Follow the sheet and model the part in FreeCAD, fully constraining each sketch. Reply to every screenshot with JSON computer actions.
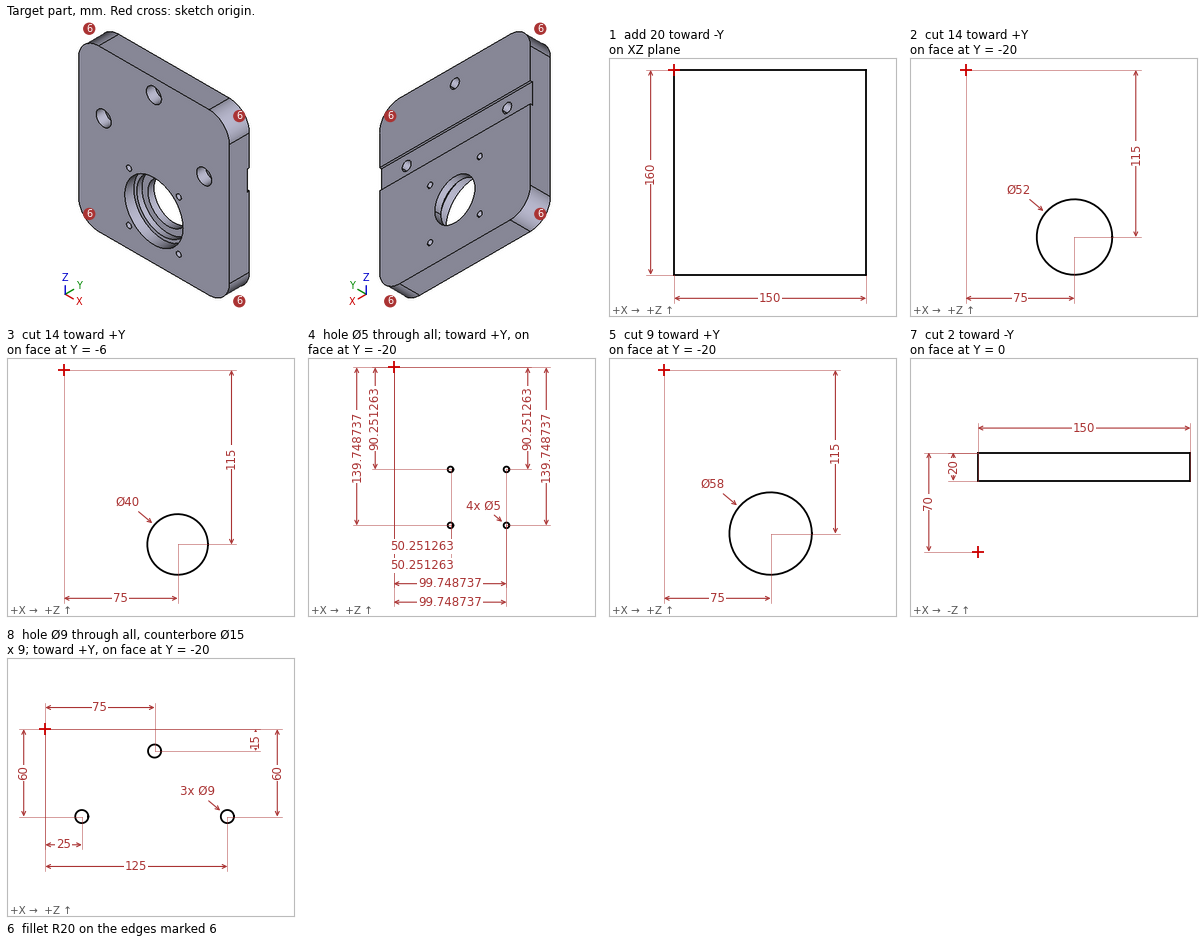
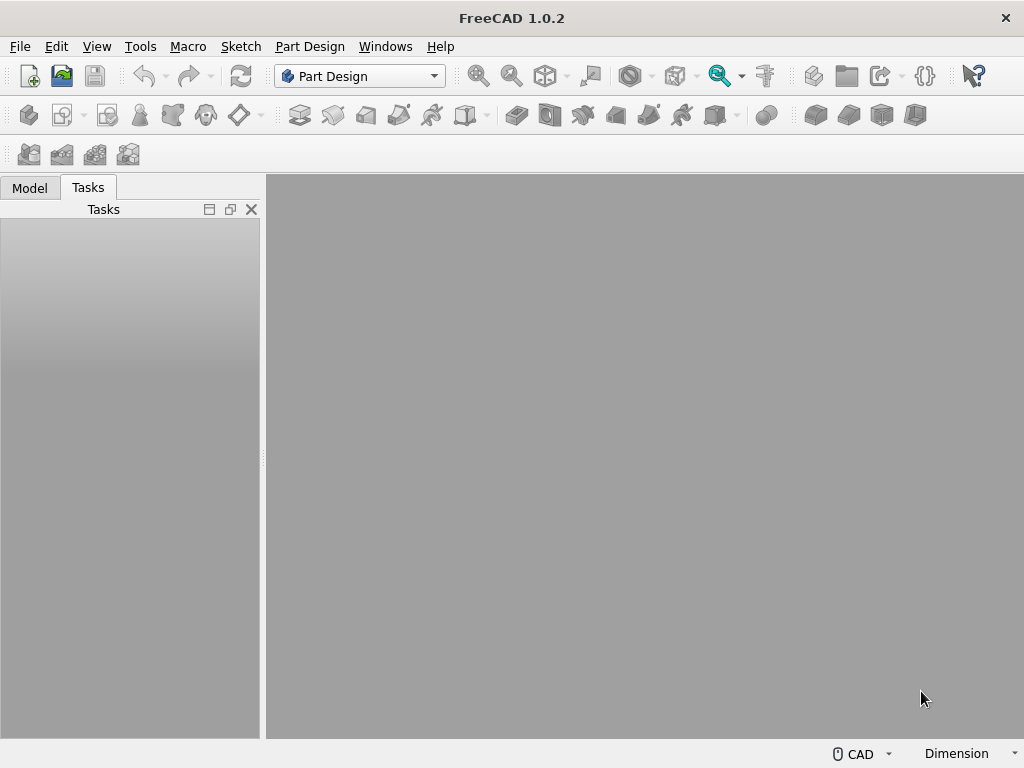
{"action": "left_click", "coordinate": [29, 76]}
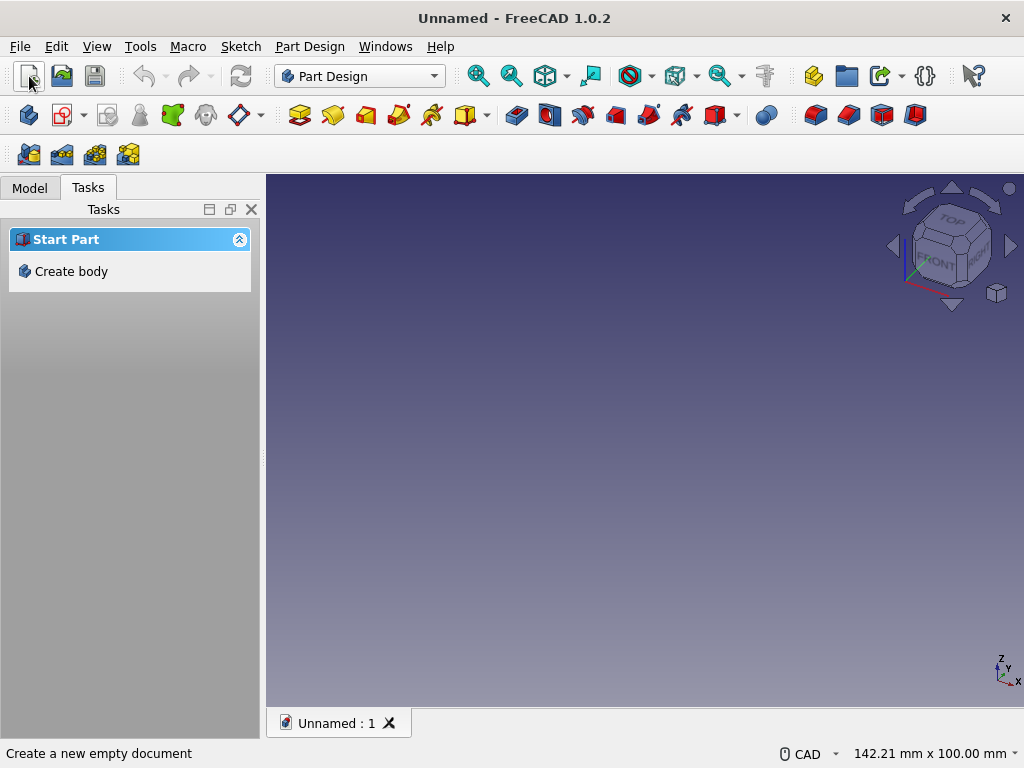
{"action": "left_click", "coordinate": [62, 116]}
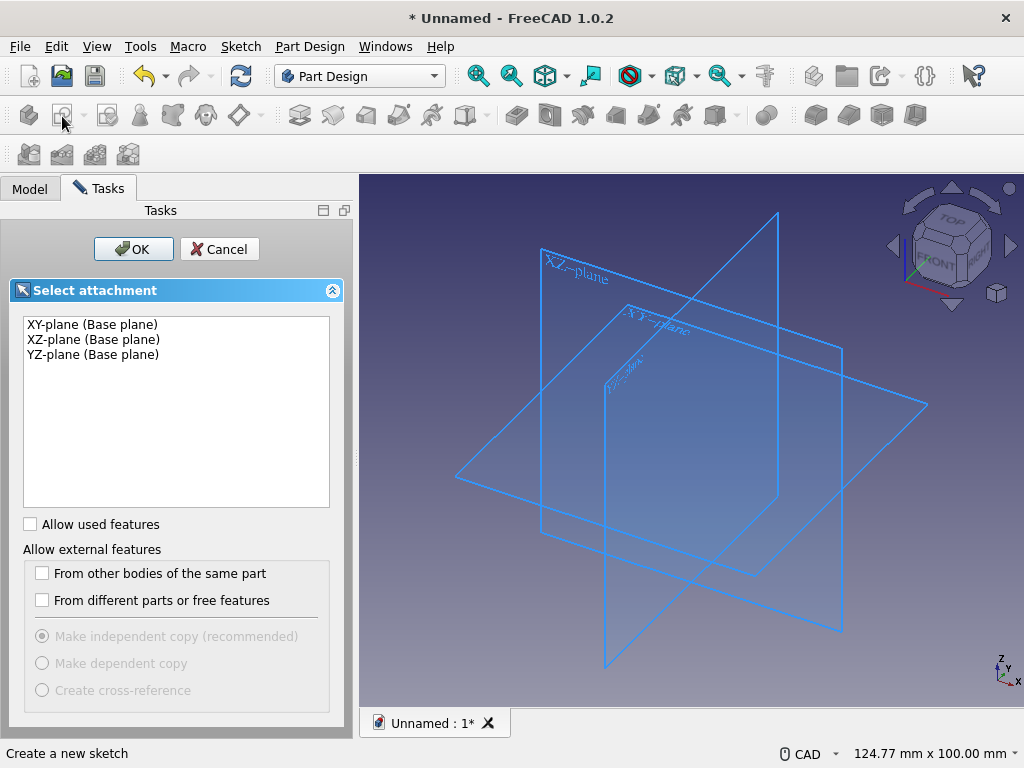
{"action": "left_click", "coordinate": [84, 340]}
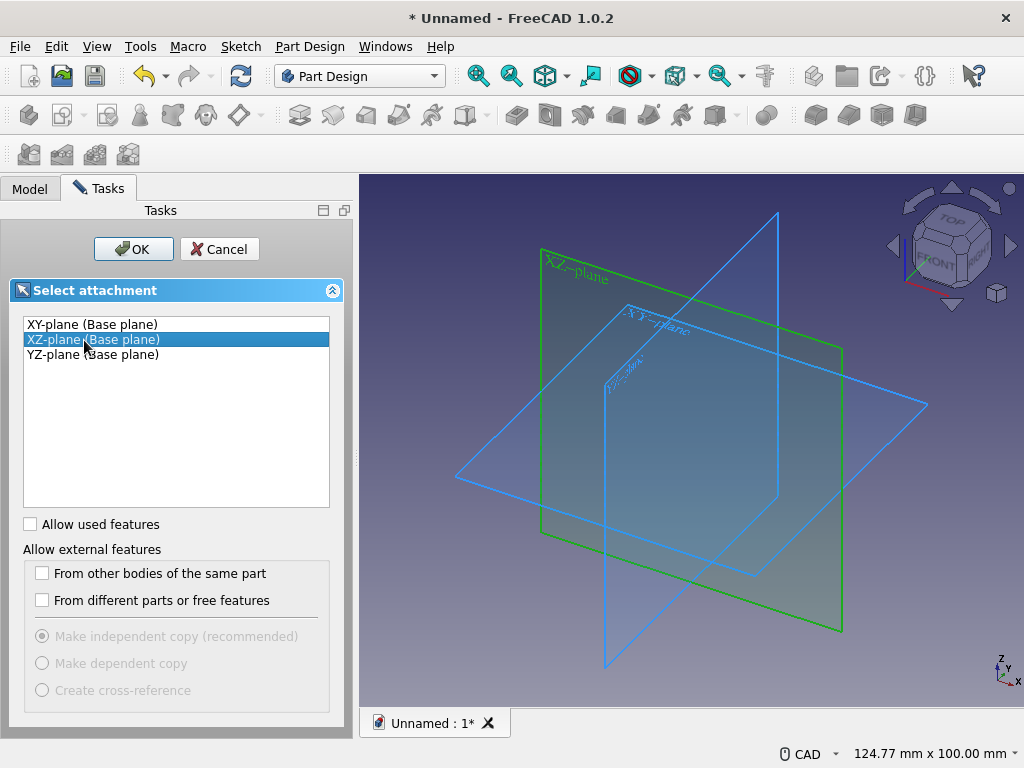
{"action": "left_click", "coordinate": [134, 249]}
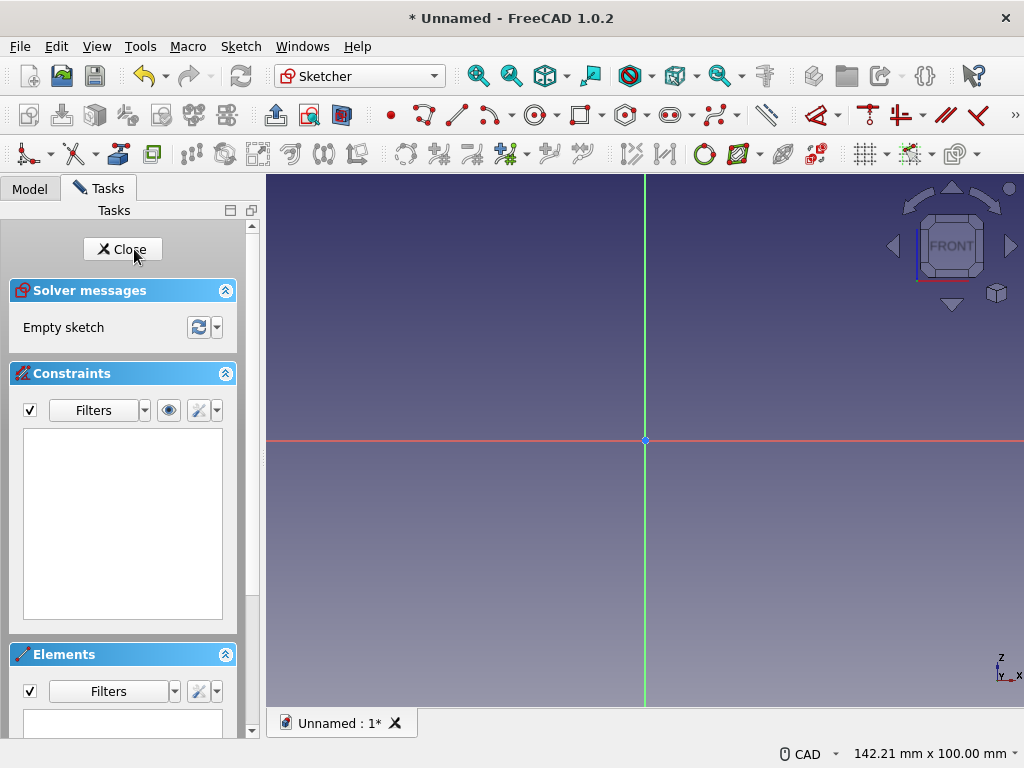
{"action": "scroll", "coordinate": [304, 202], "scroll_direction": "down", "scroll_amount": 5}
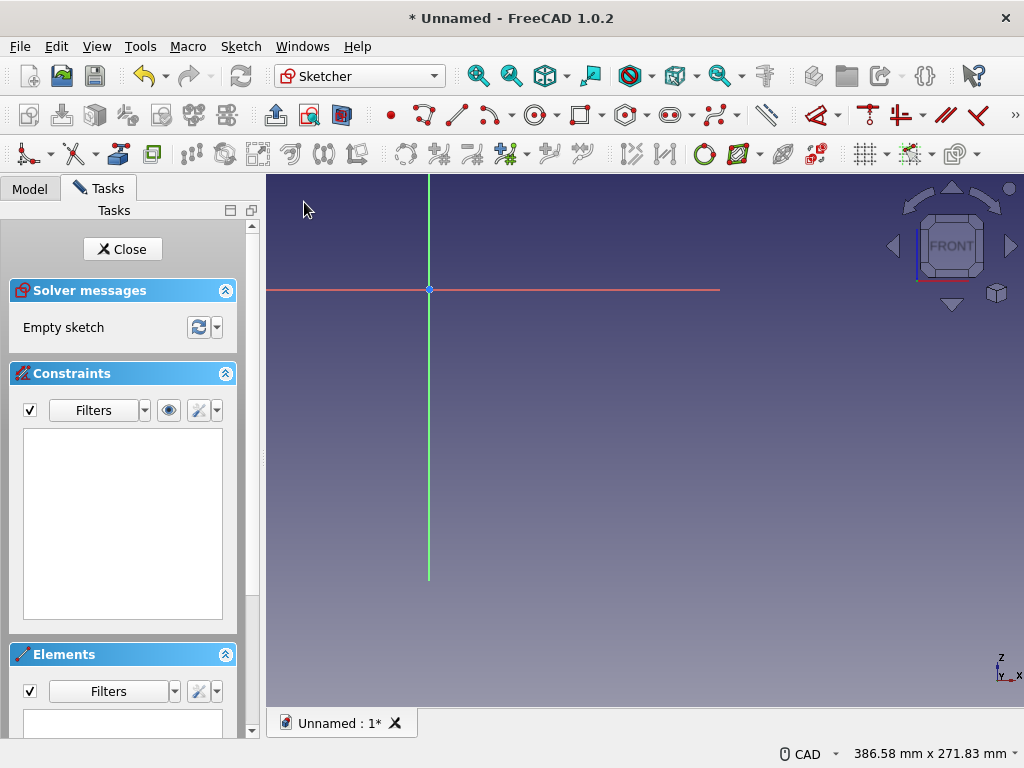
{"action": "left_click", "coordinate": [580, 116]}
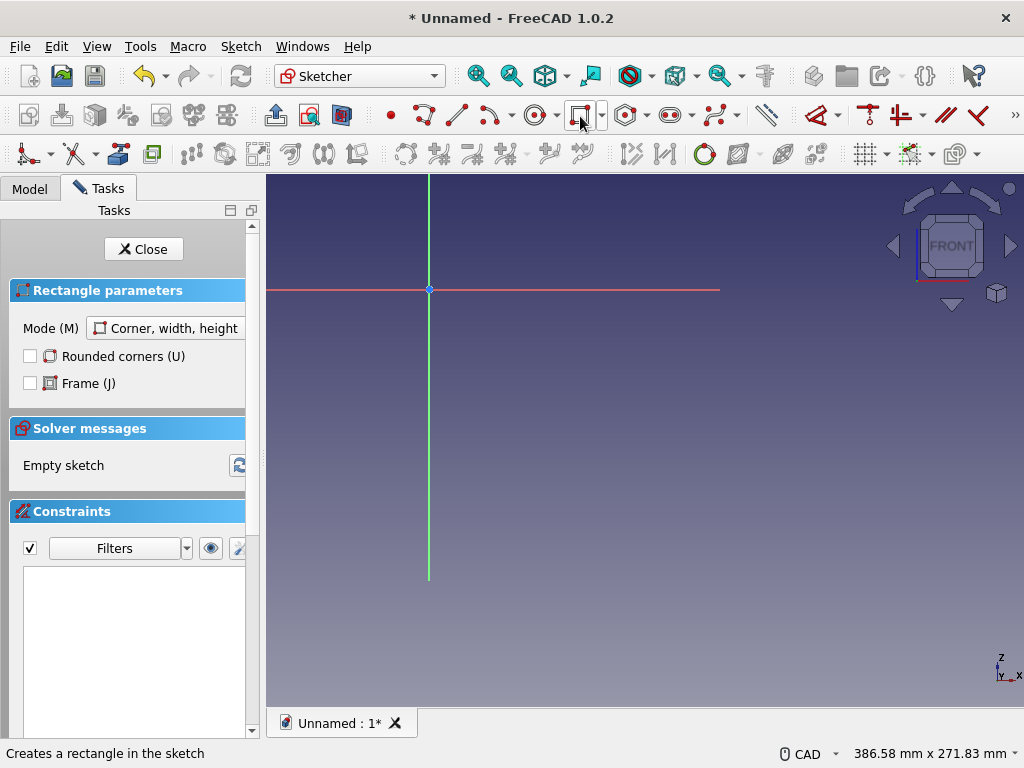
{"action": "left_click", "coordinate": [429, 290]}
{"action": "left_click", "coordinate": [724, 604]}
{"action": "key", "text": "Escape"}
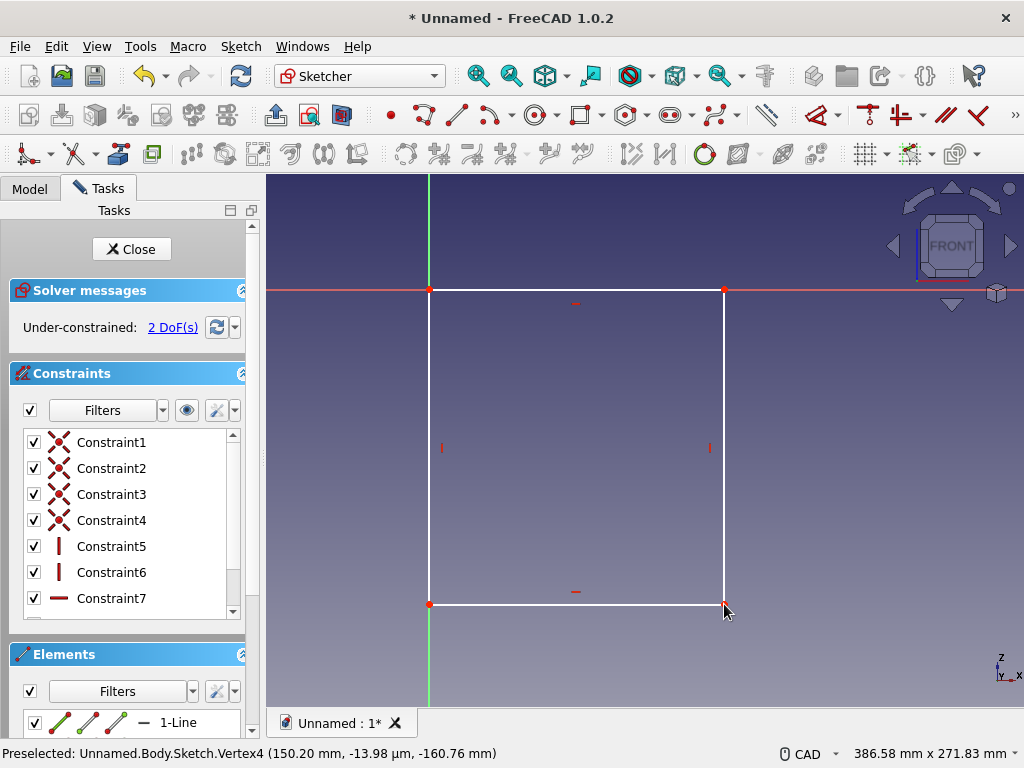
{"action": "left_click", "coordinate": [429, 384]}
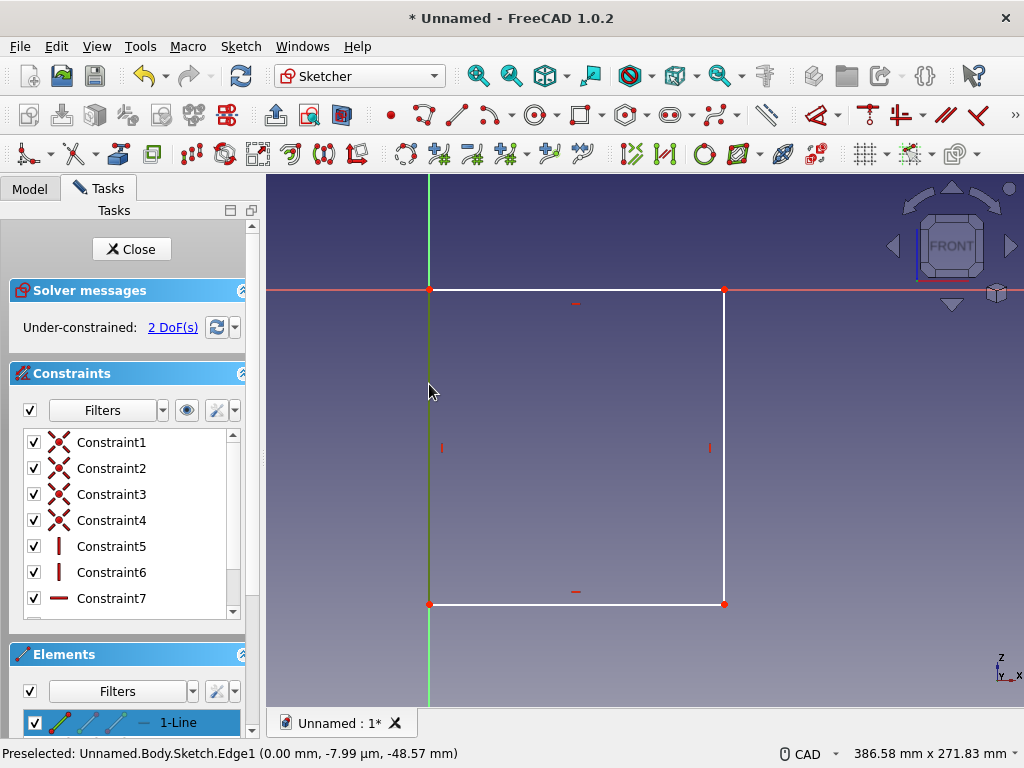
{"action": "key", "text": "i"}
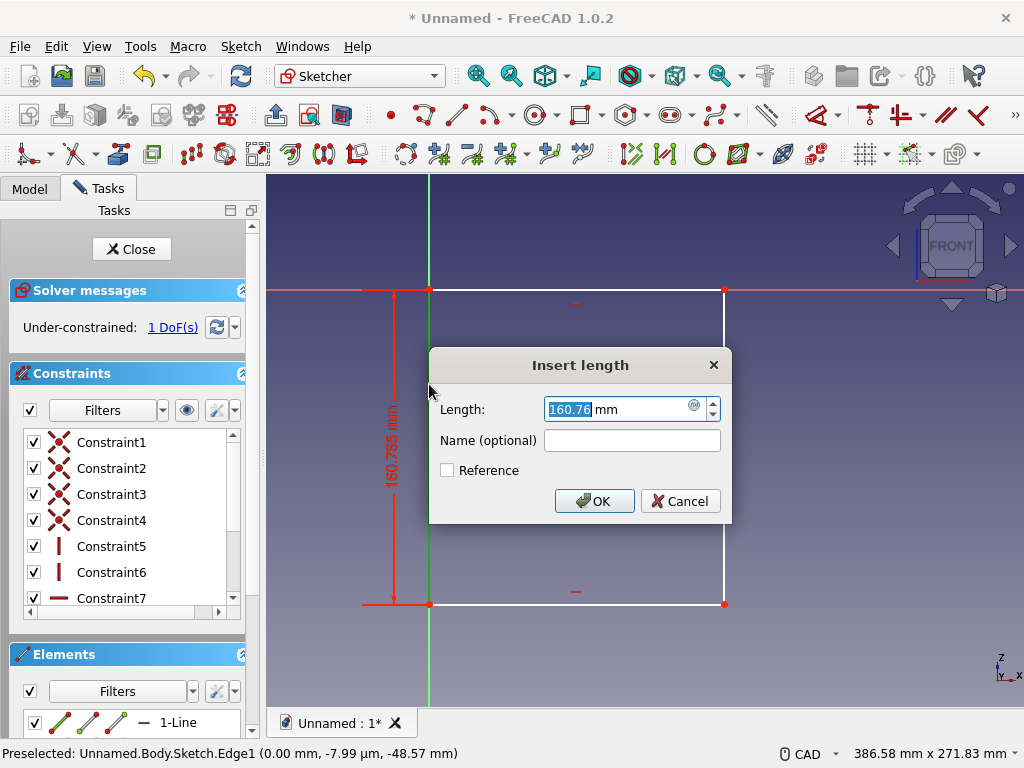
{"action": "type", "text": "160"}
{"action": "key", "text": "Return"}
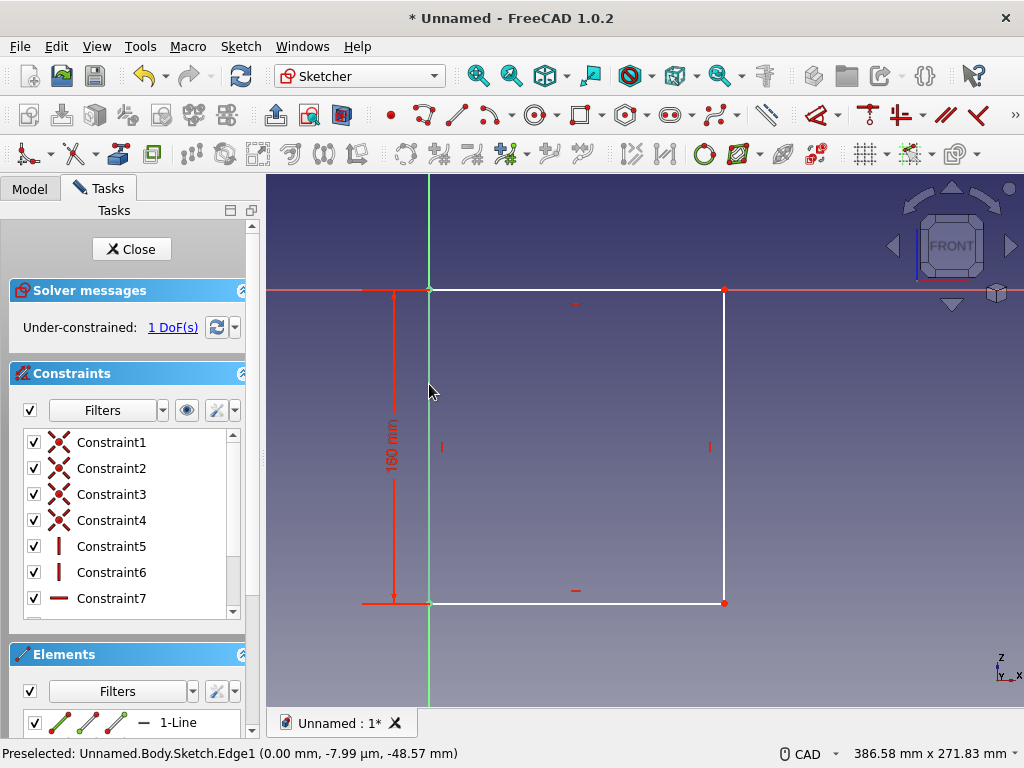
{"action": "left_click", "coordinate": [518, 604]}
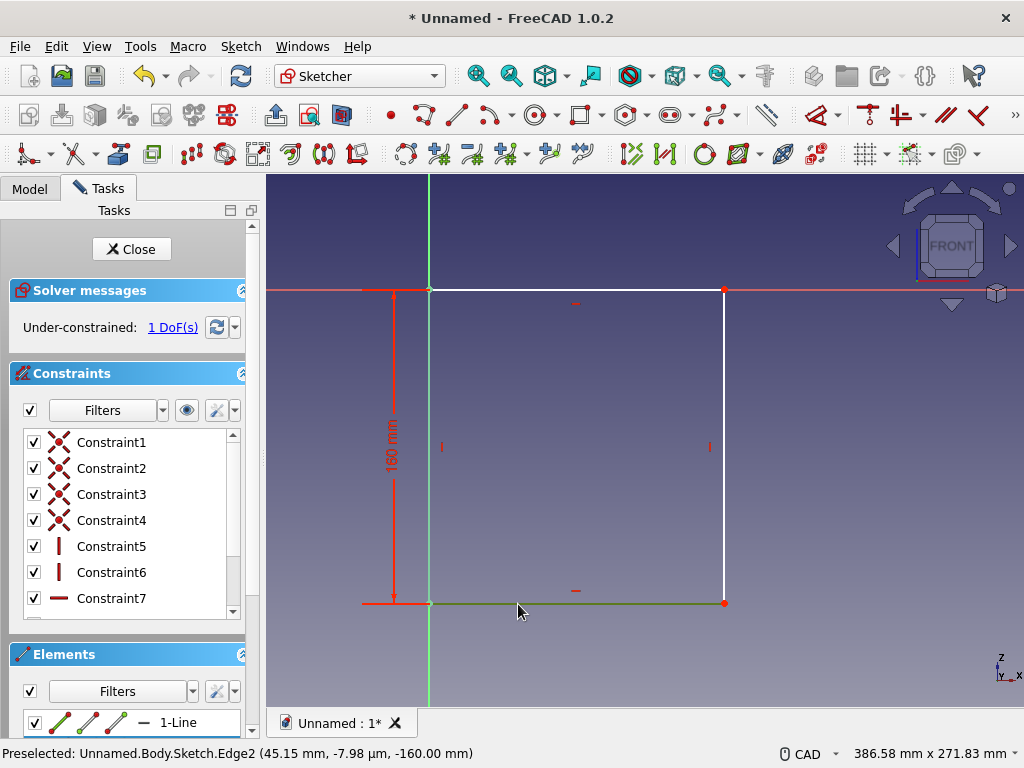
{"action": "key", "text": "l"}